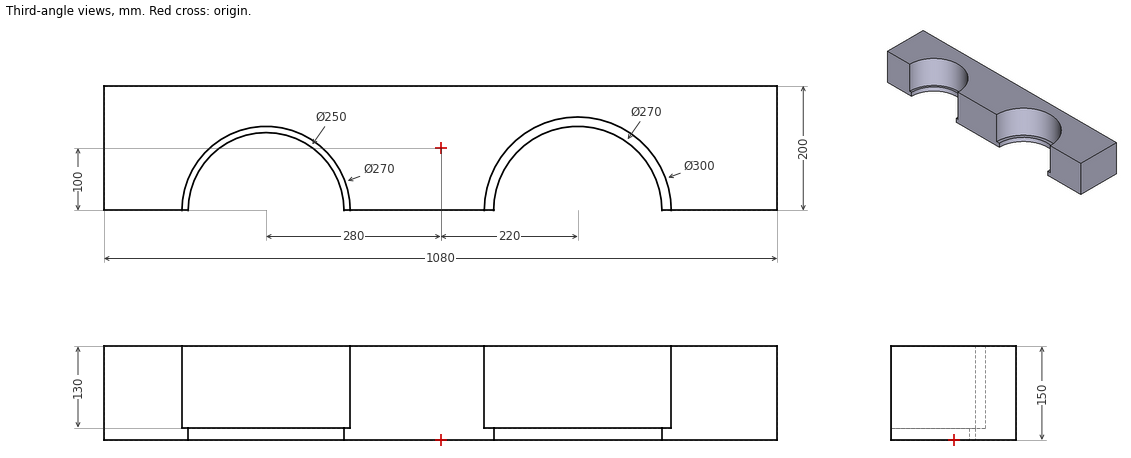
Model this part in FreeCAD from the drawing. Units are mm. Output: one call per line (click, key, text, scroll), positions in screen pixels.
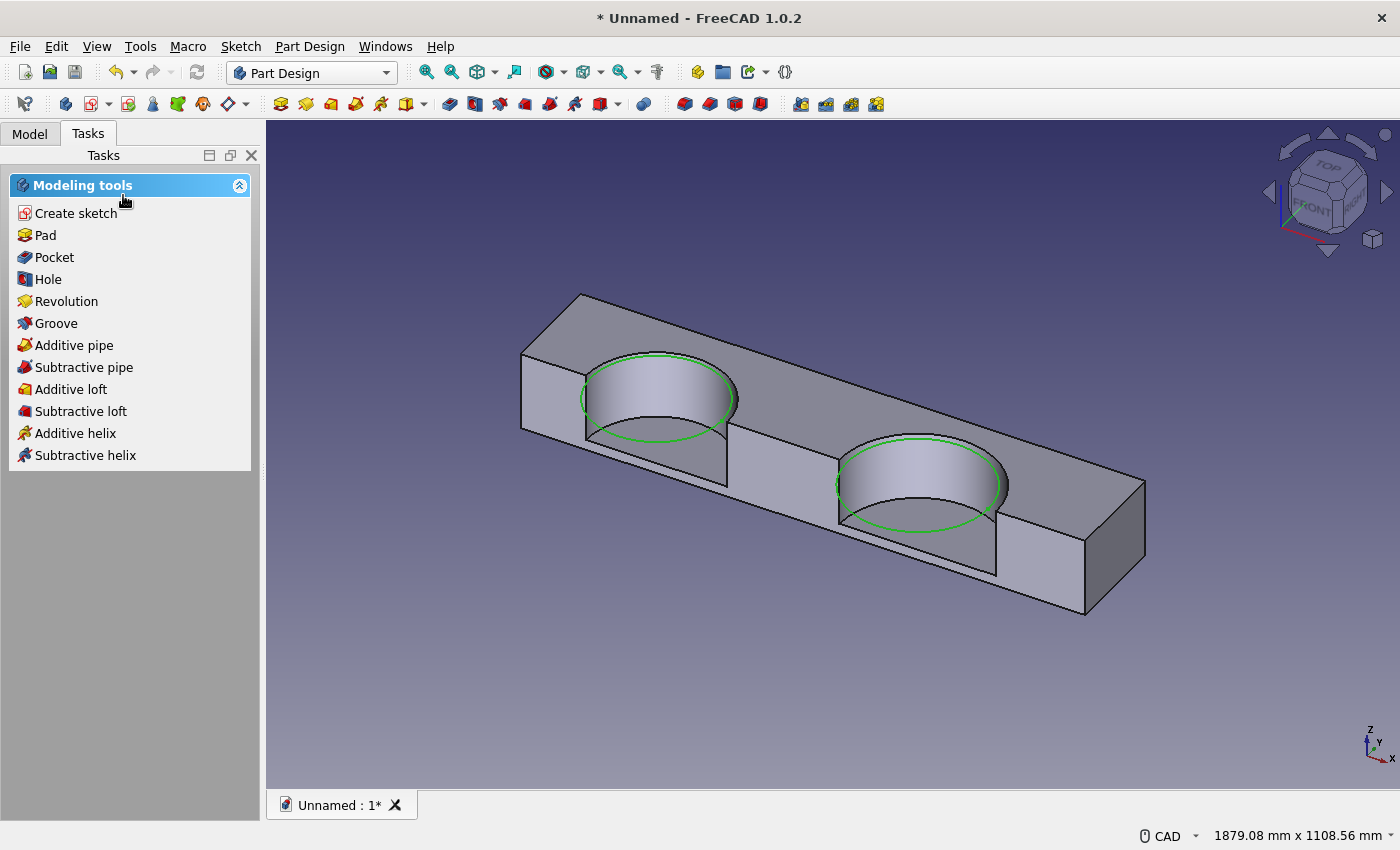
click(450, 104)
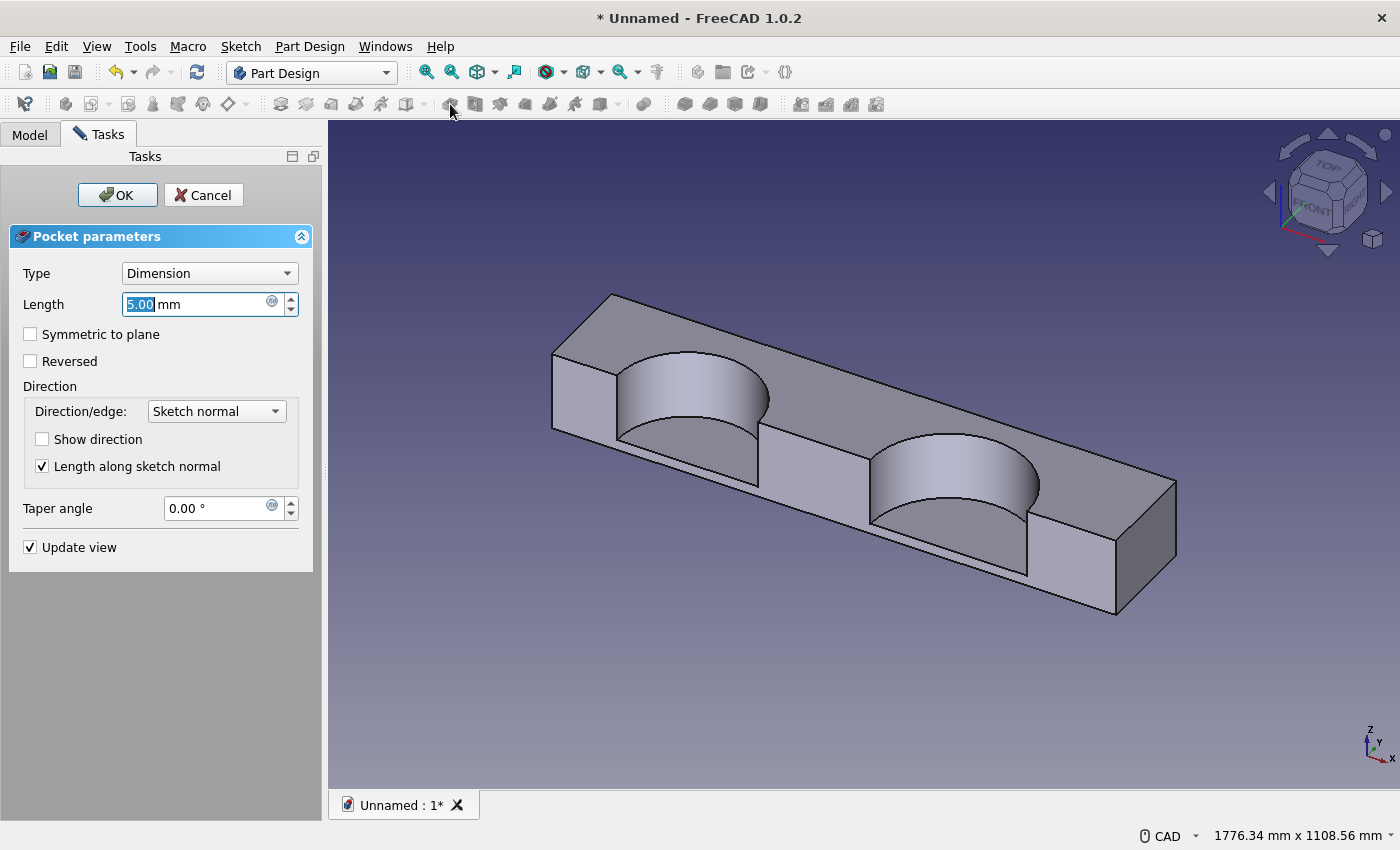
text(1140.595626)
key(Tab)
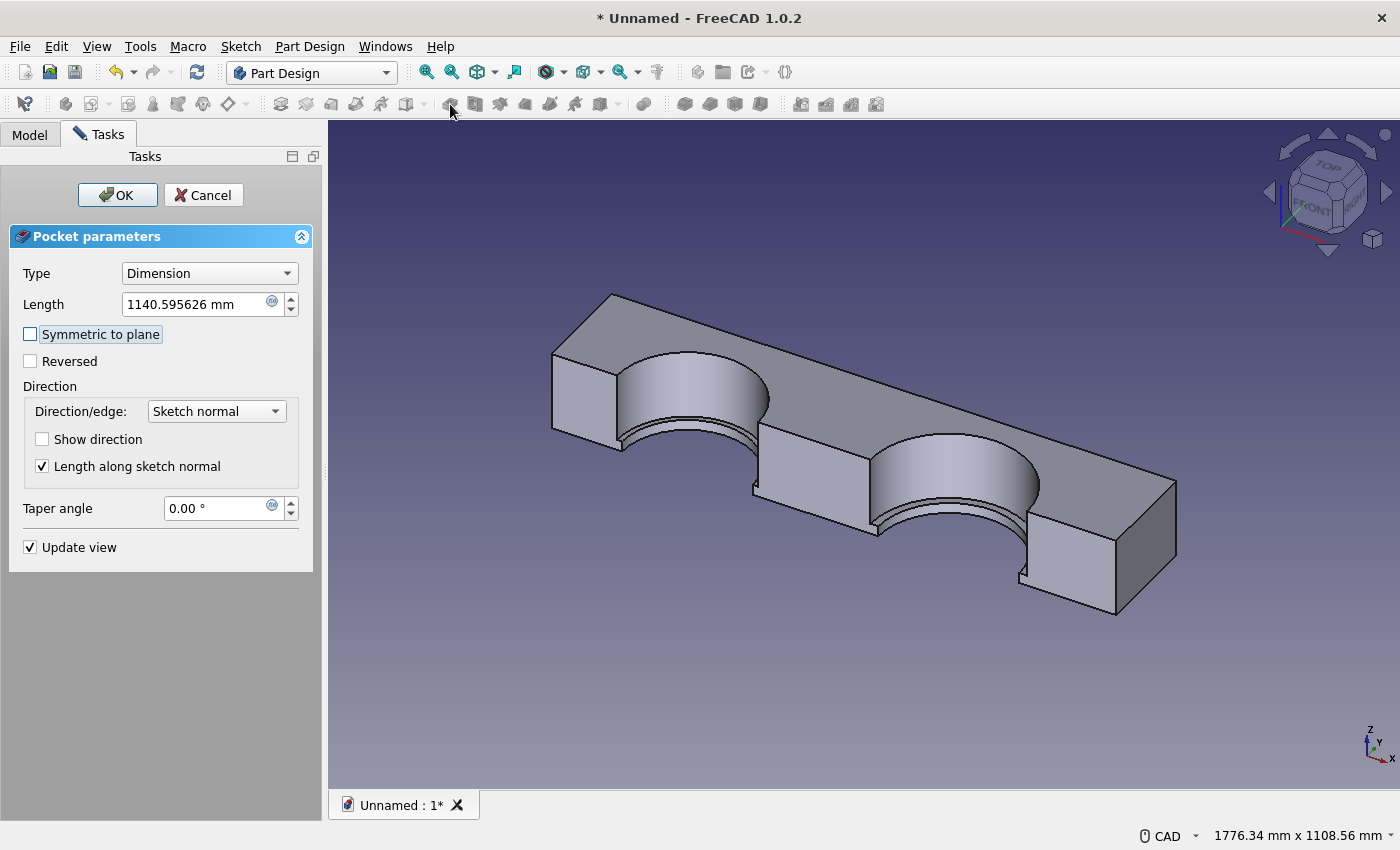
click(31, 334)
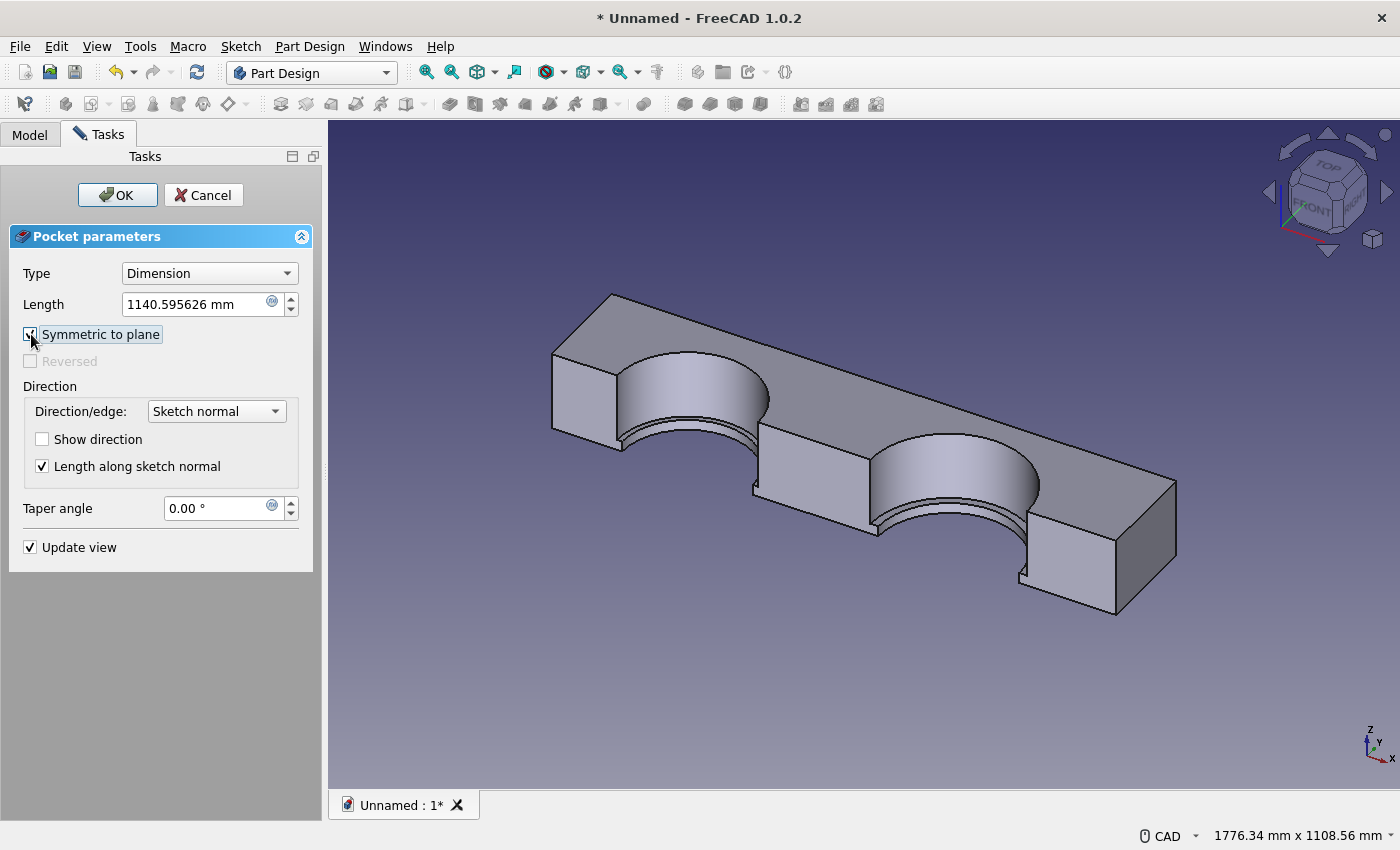
click(118, 195)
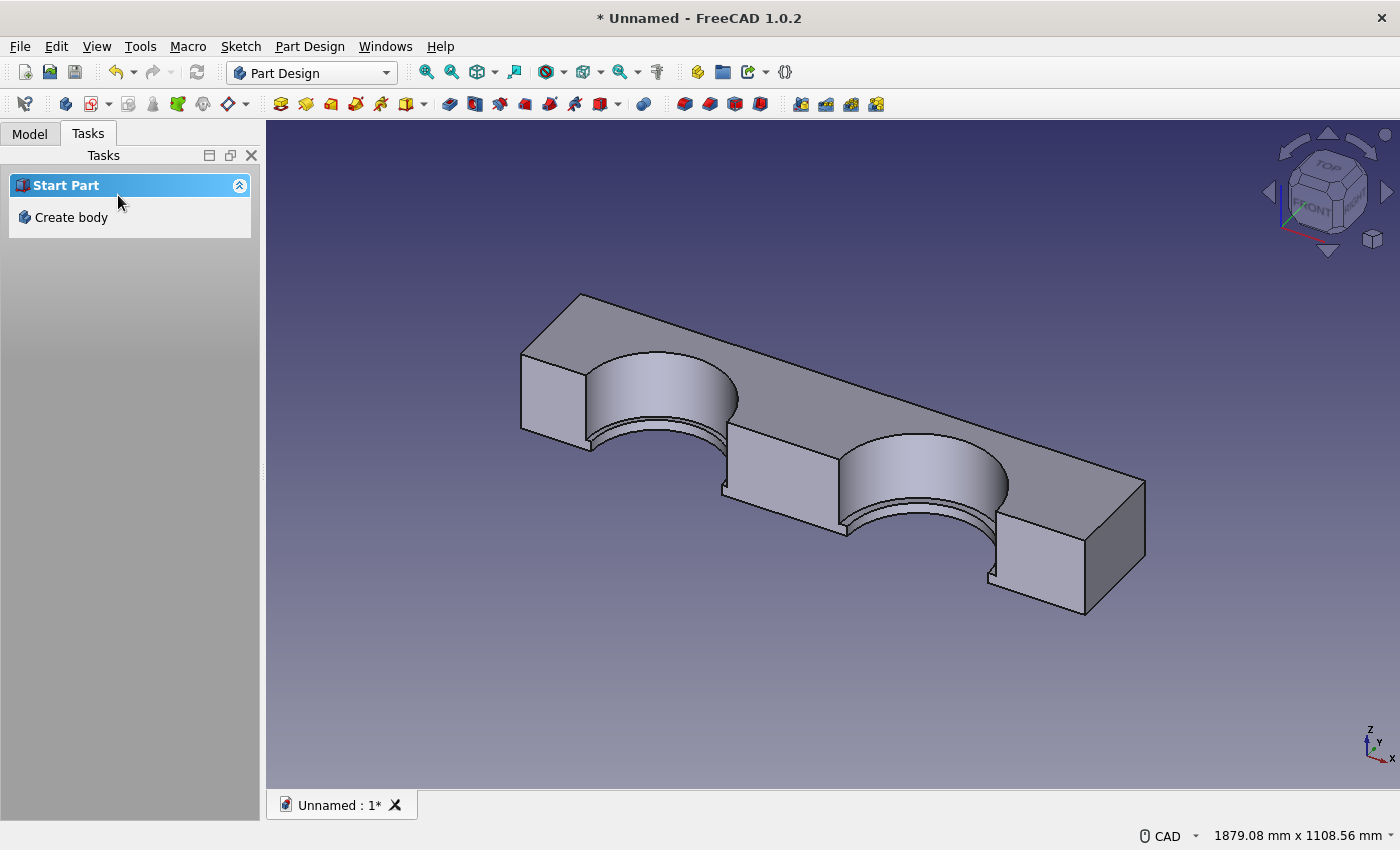
key(0)